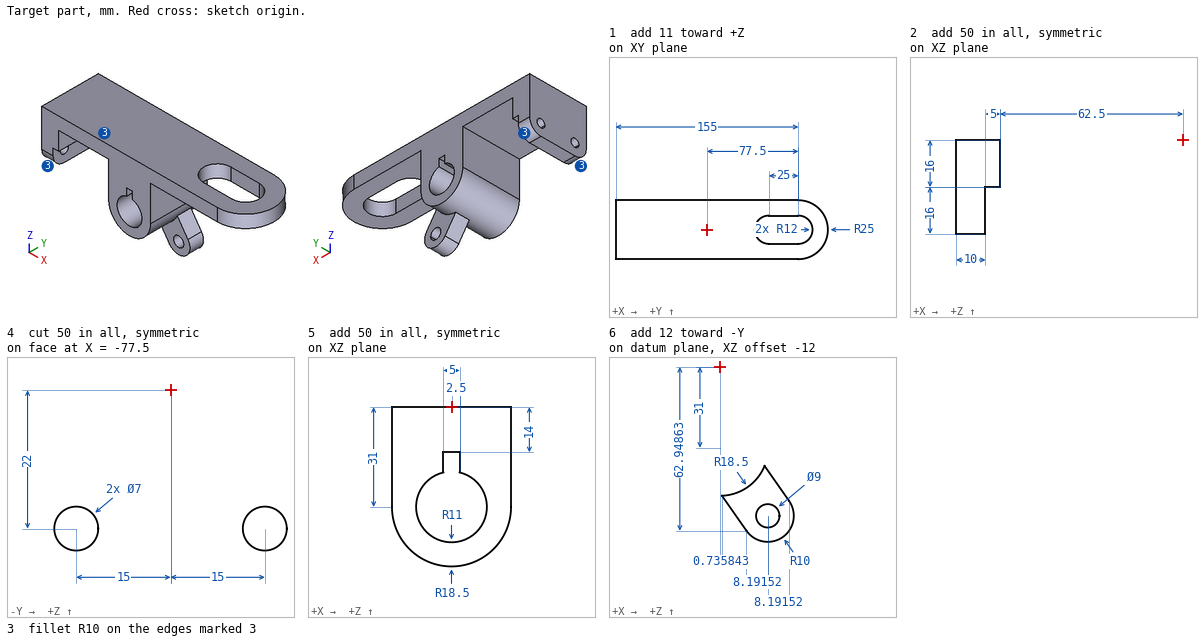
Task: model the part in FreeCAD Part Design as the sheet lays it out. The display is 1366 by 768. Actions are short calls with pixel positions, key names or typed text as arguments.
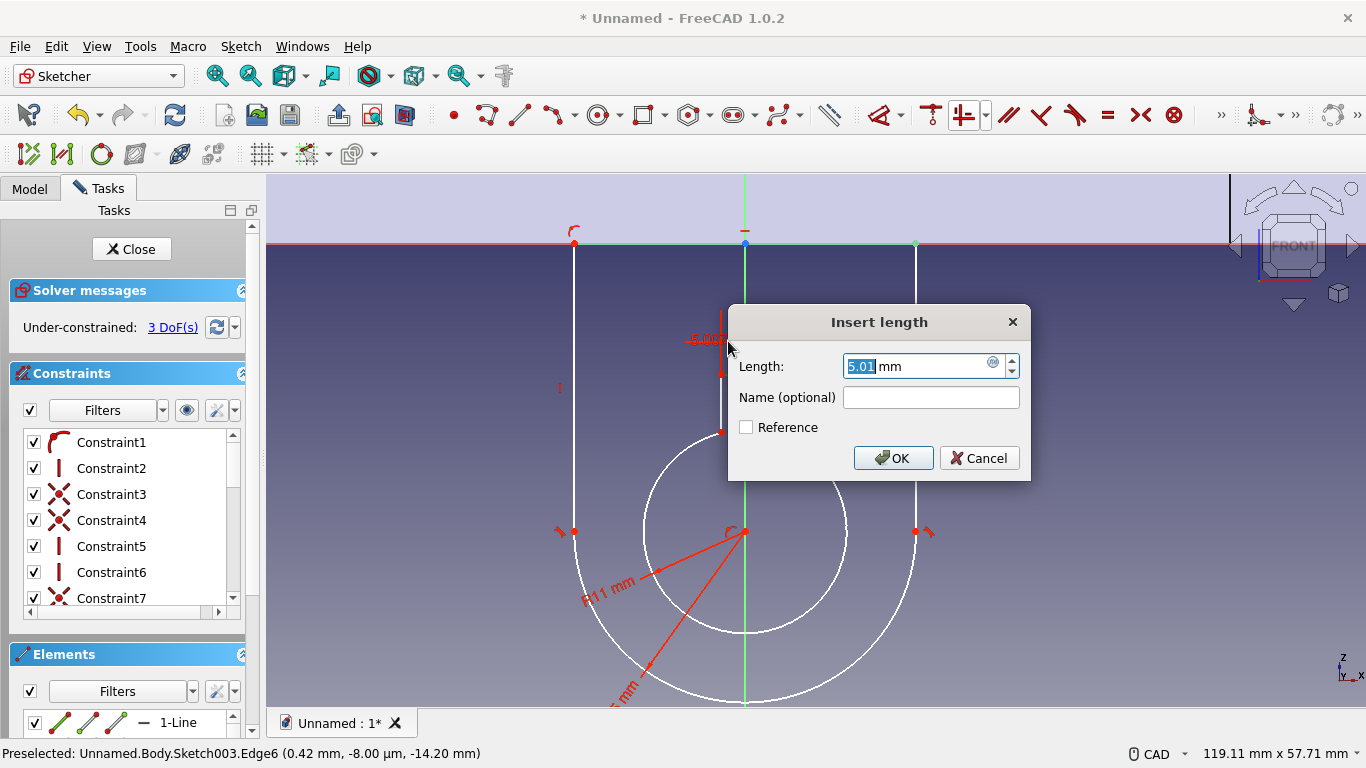
text(5)
key(Return)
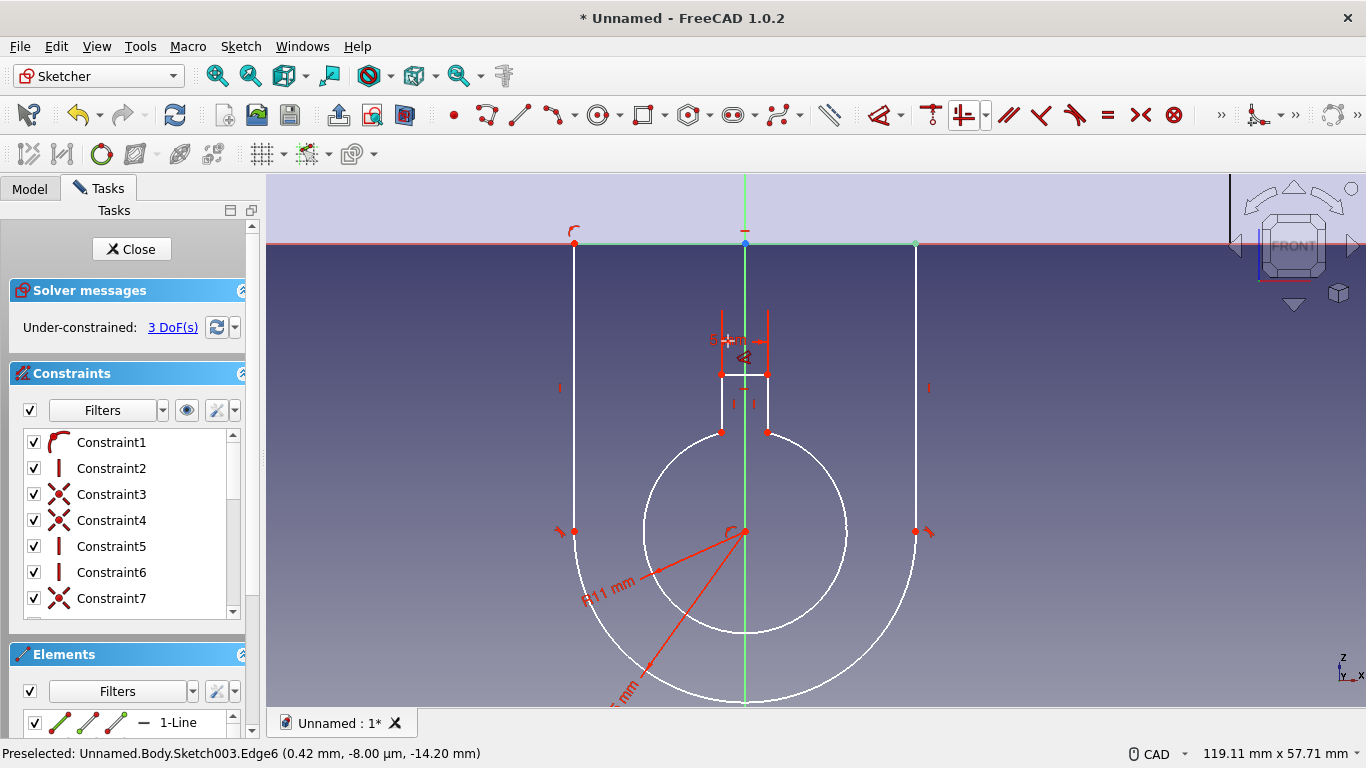
click(574, 445)
click(540, 388)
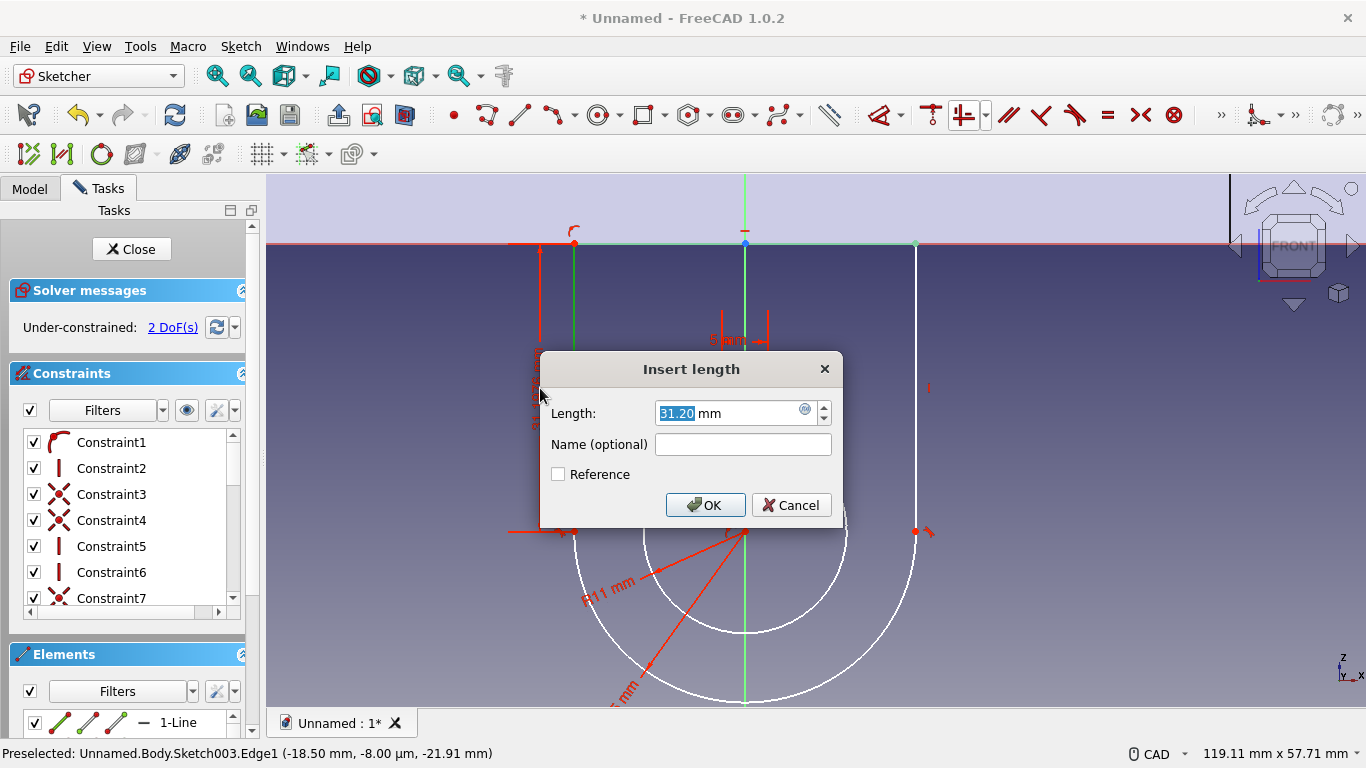
text(31)
key(Return)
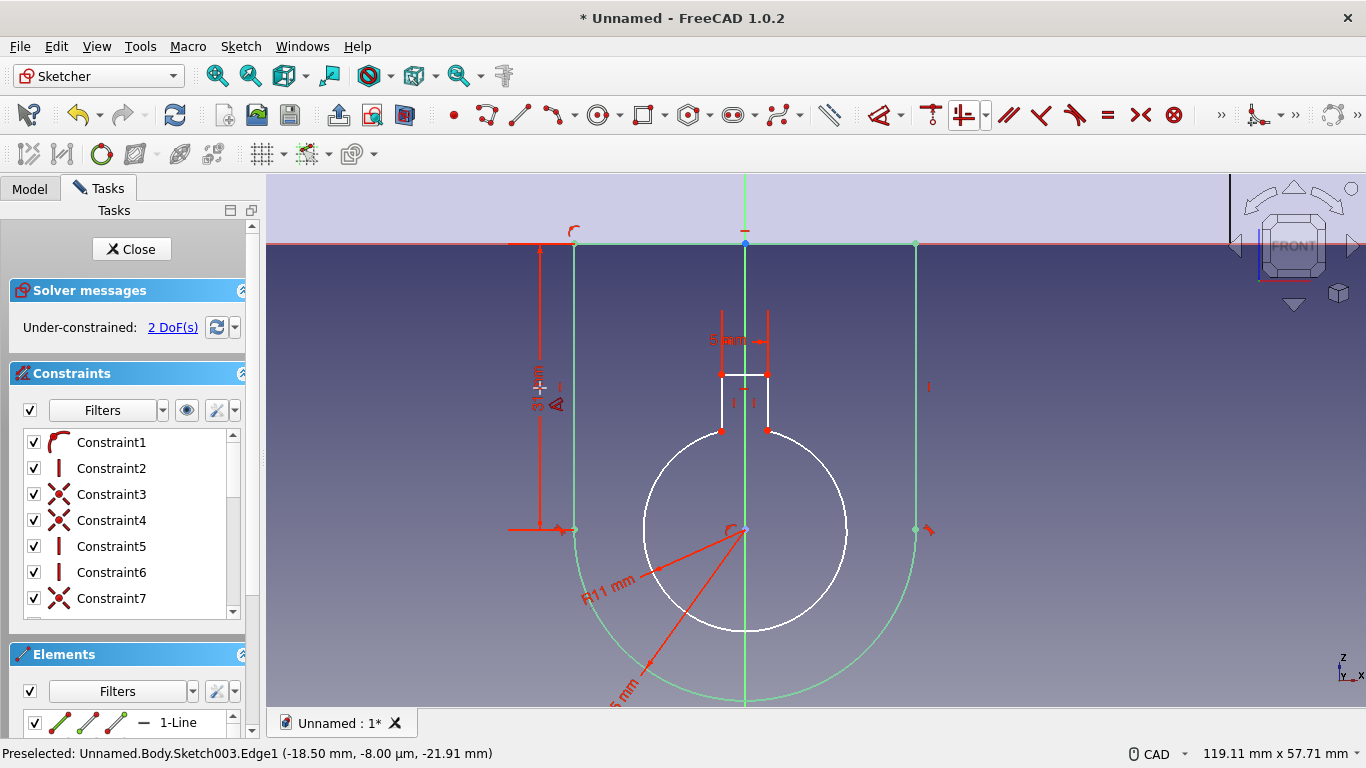
click(768, 375)
click(802, 309)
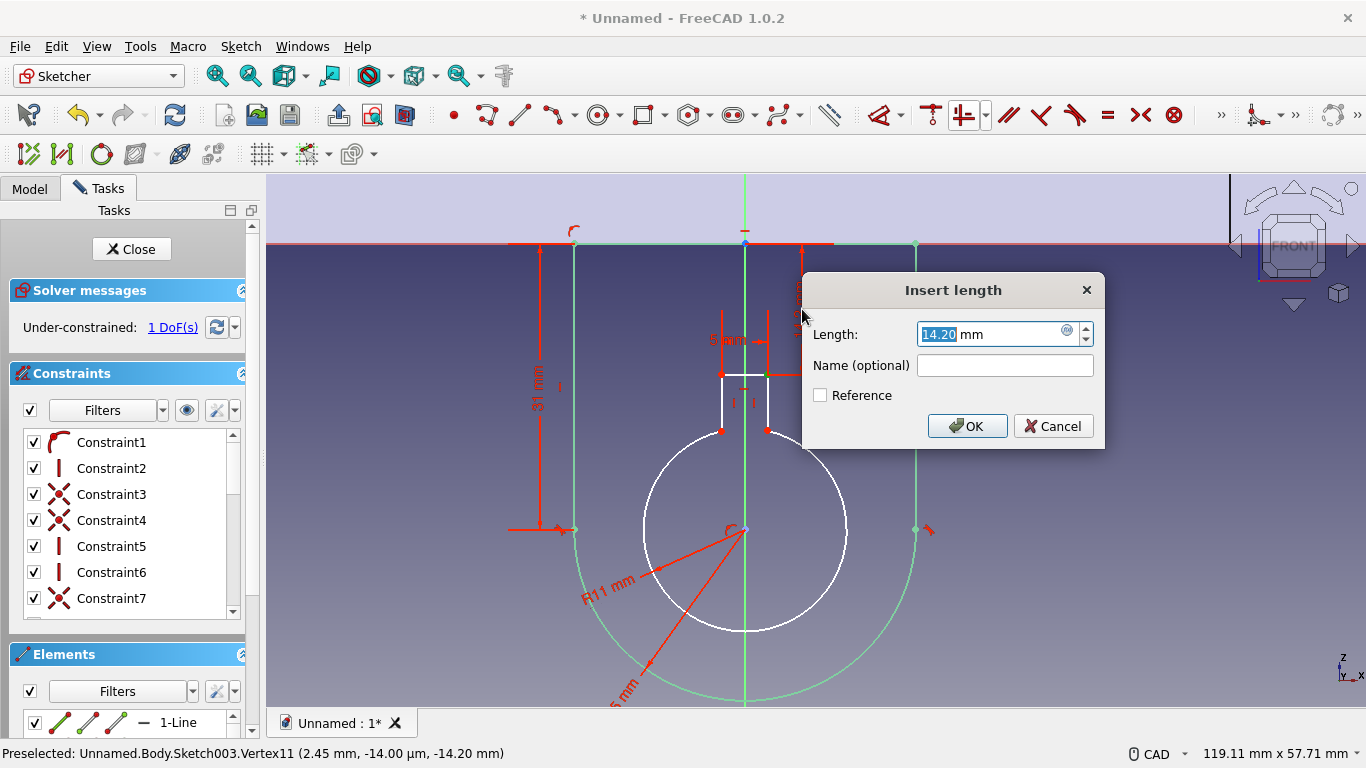
text(14)
key(Return)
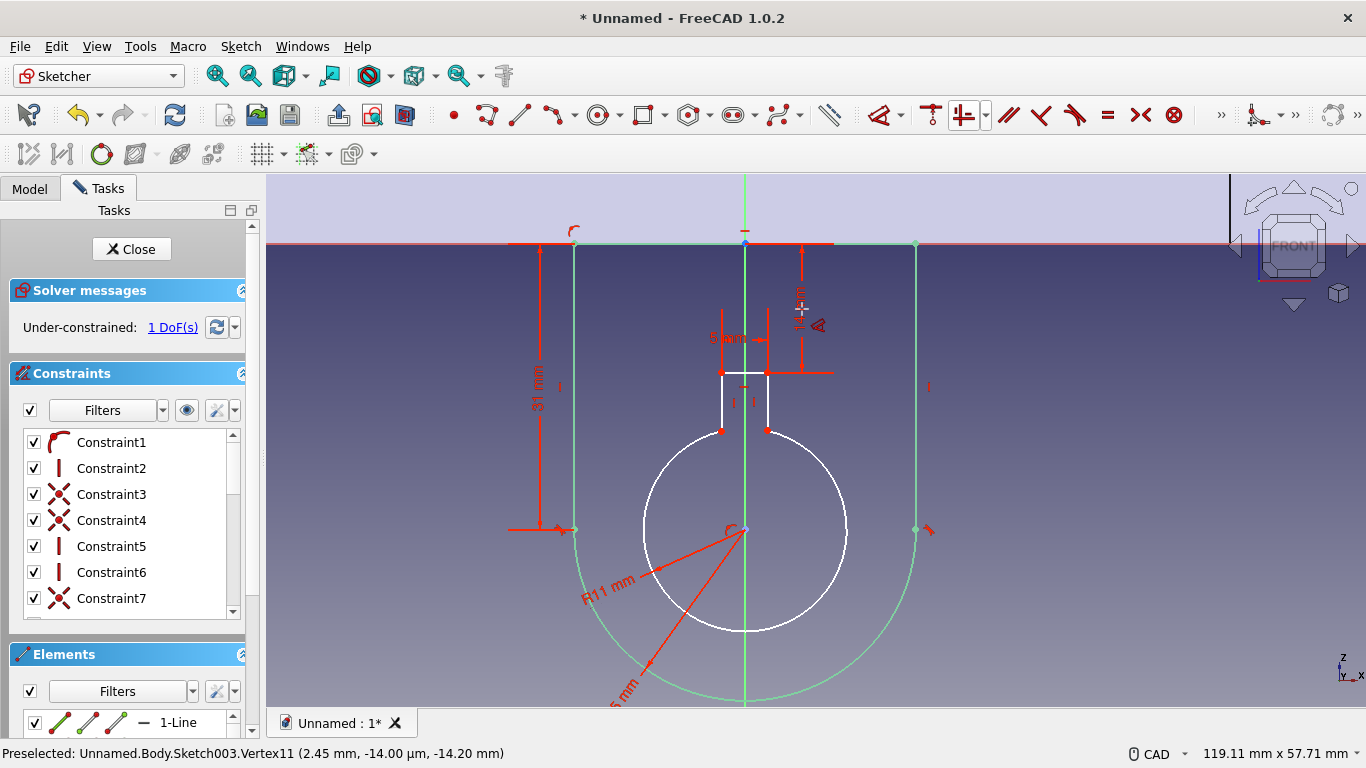
scroll(768, 431, up, 3)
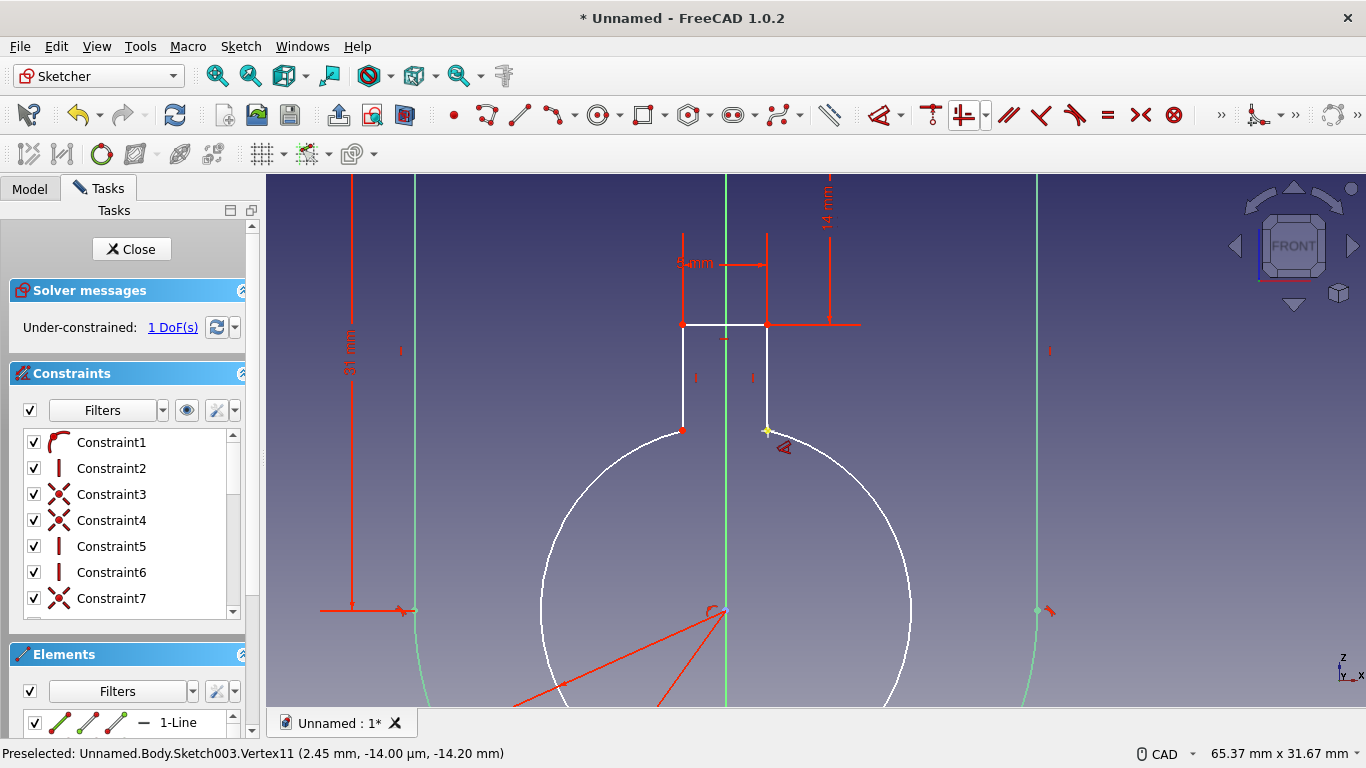
click(767, 430)
click(746, 464)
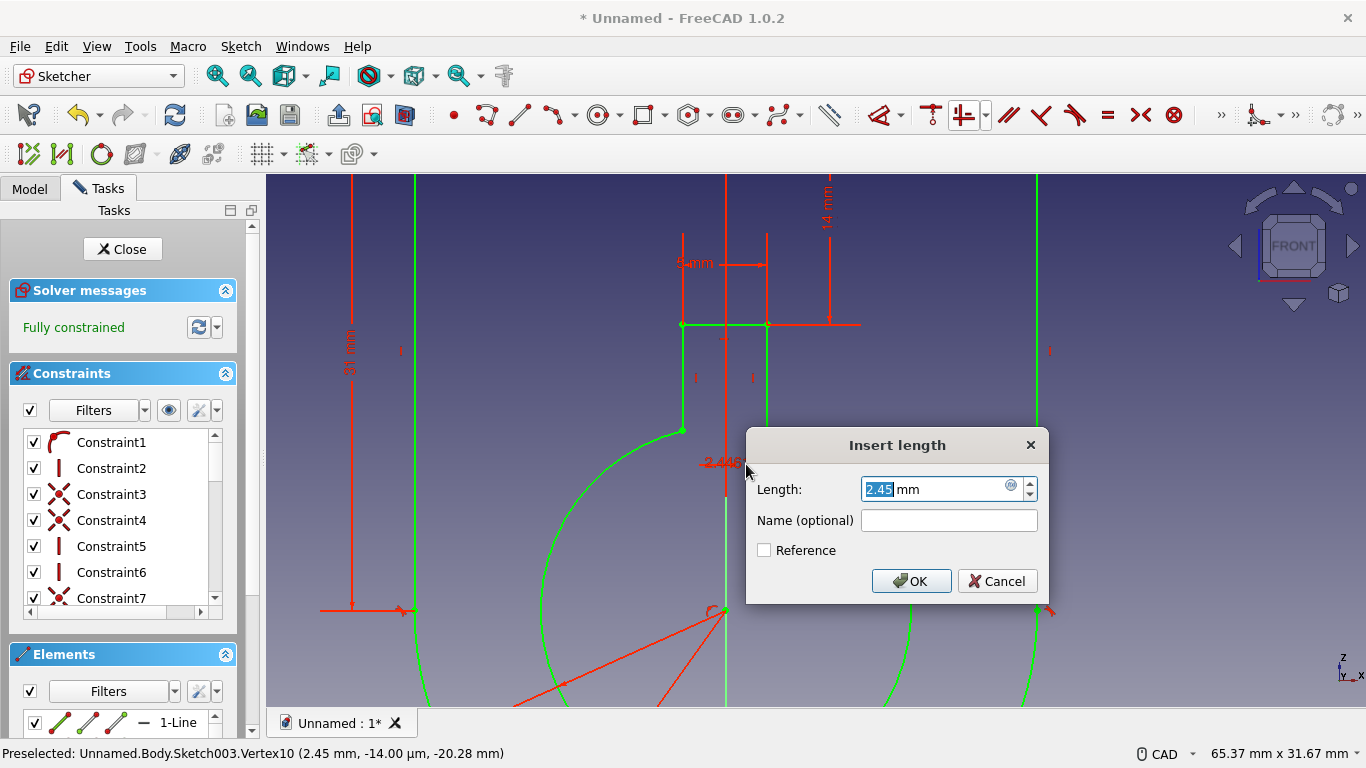
text(2.5)
key(Return)
key(Escape)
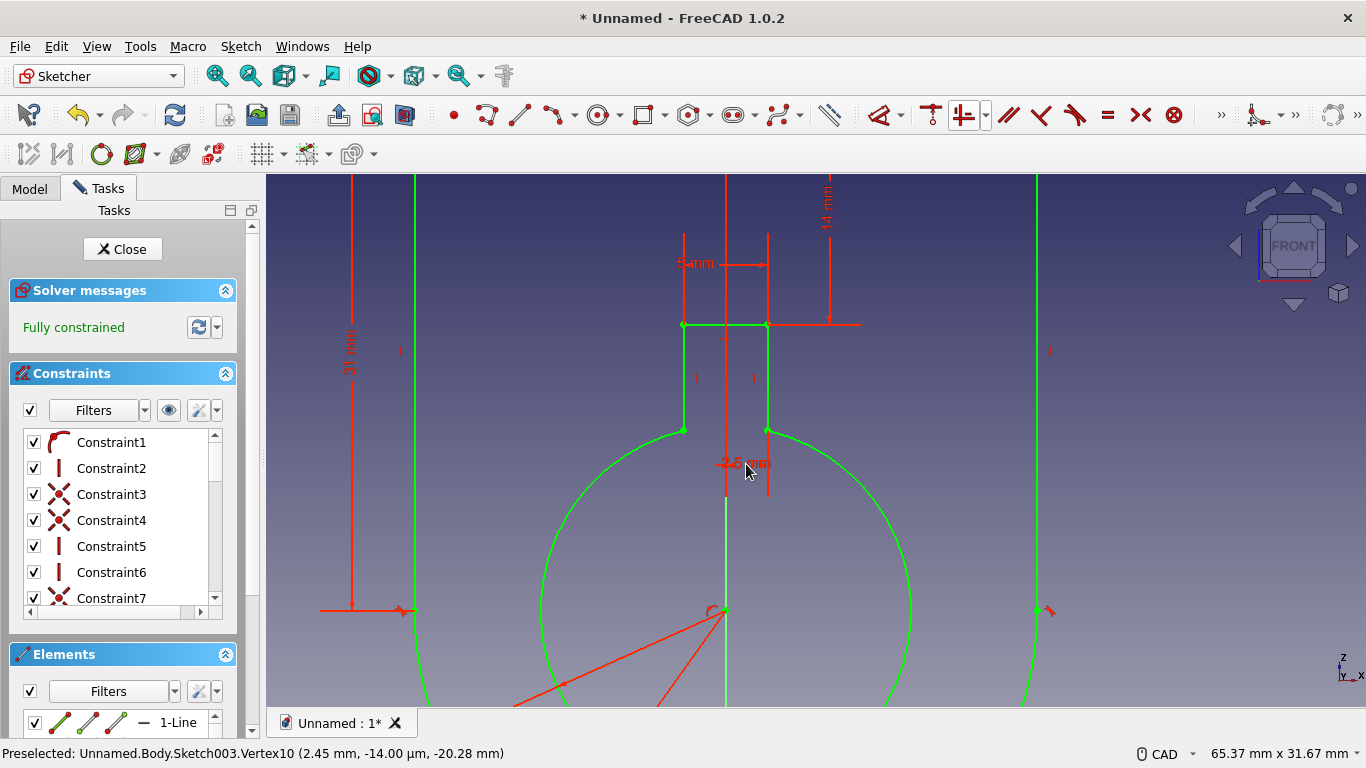
click(123, 249)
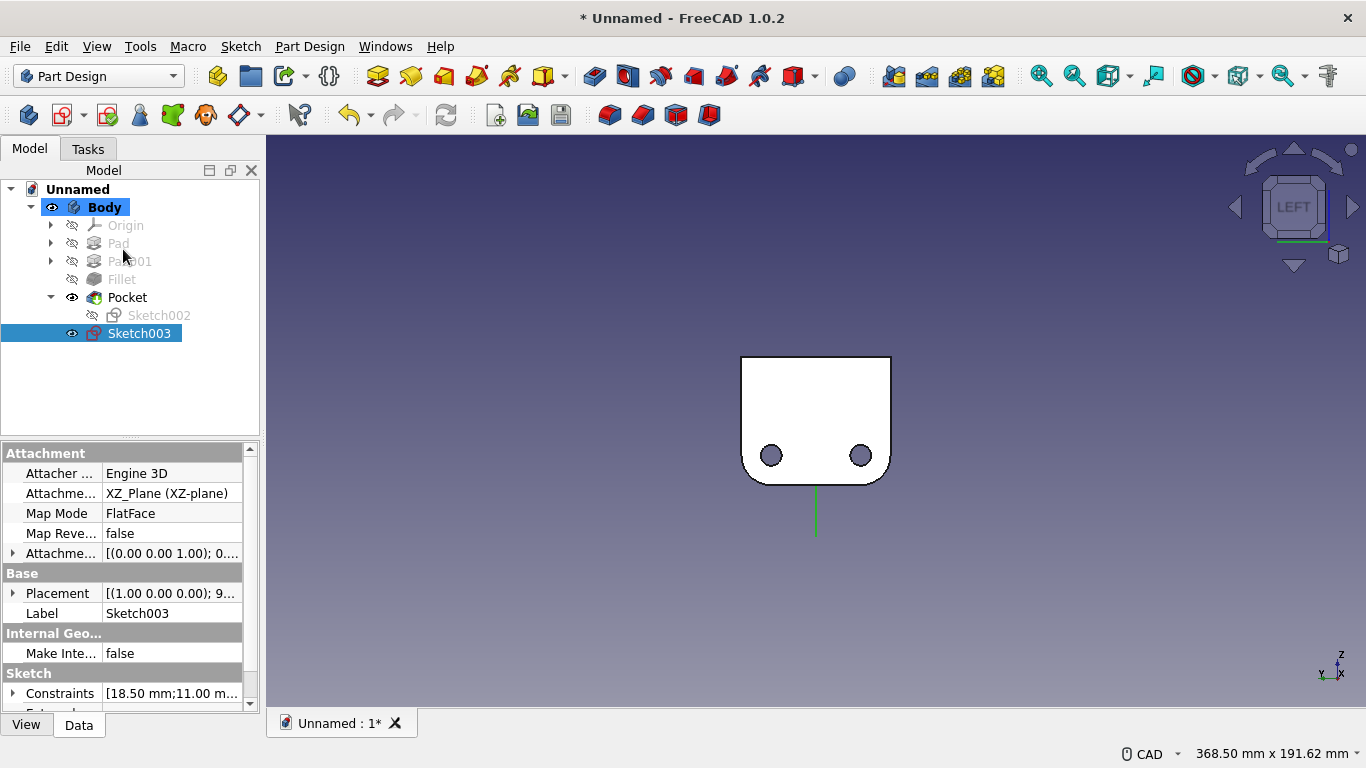
click(378, 76)